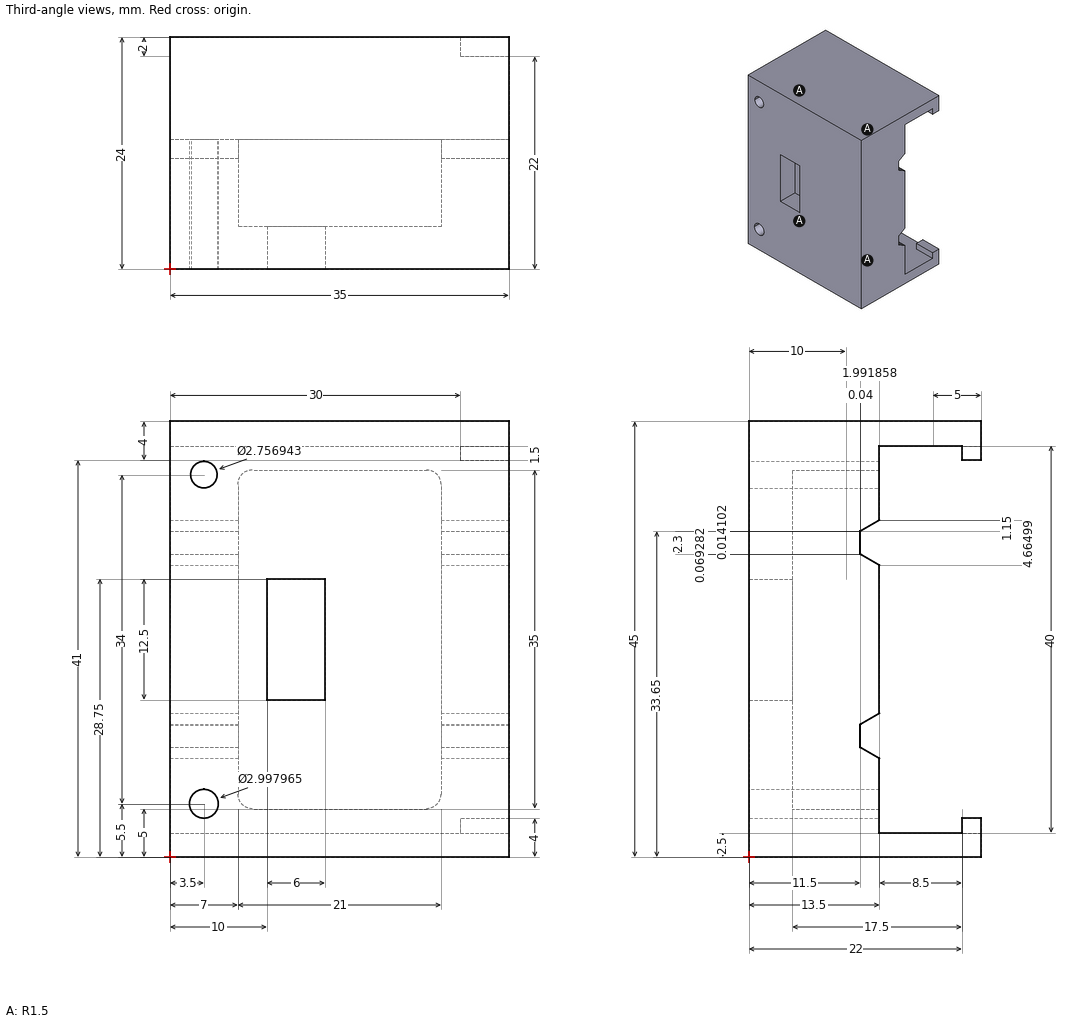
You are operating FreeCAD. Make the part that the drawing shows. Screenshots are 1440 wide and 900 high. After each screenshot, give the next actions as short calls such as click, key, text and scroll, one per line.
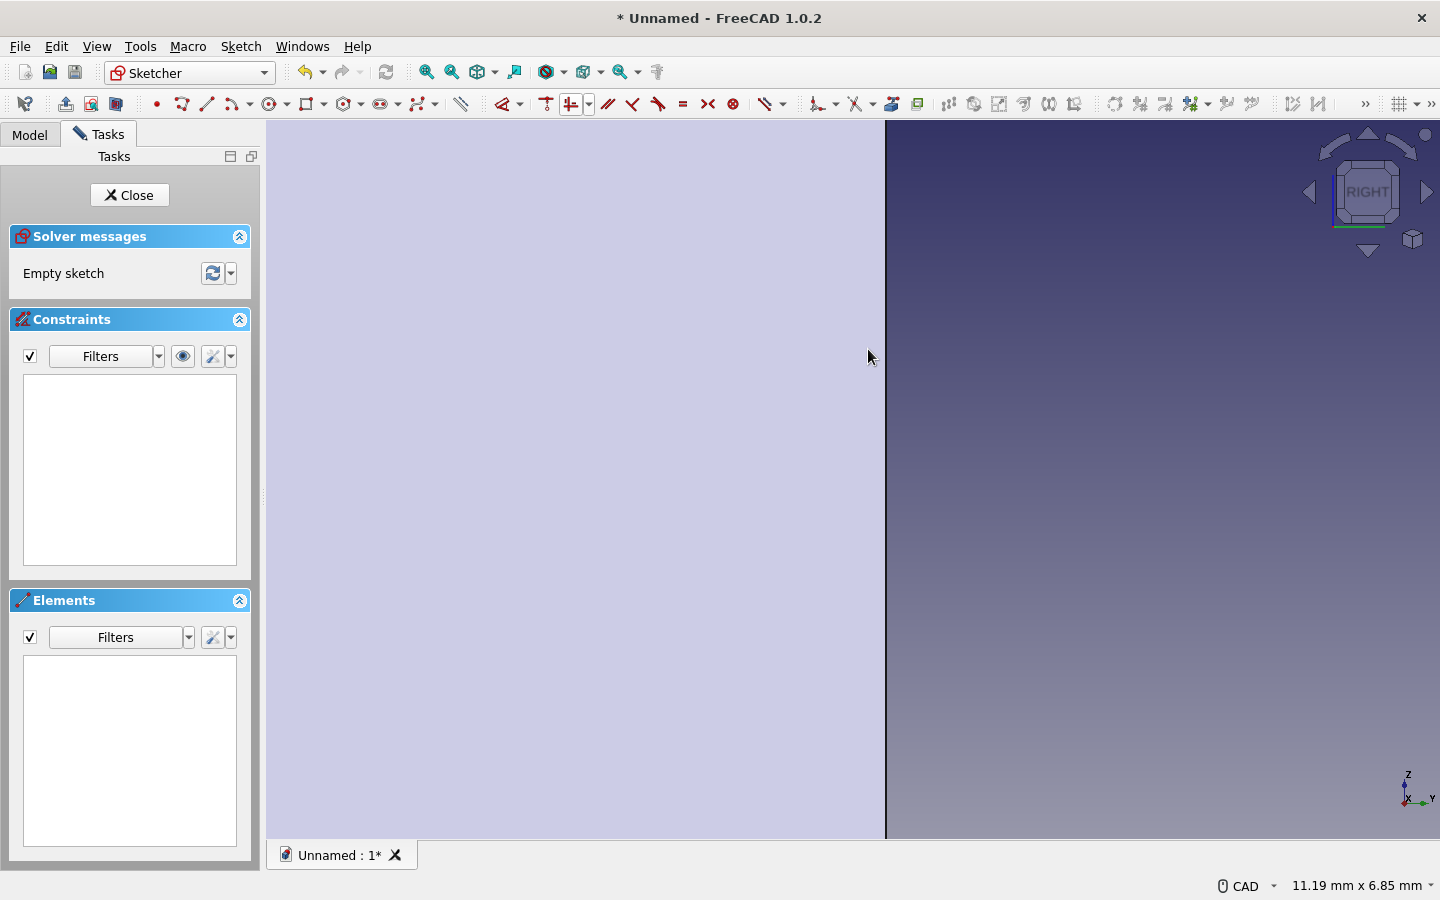
key(g)
key(m)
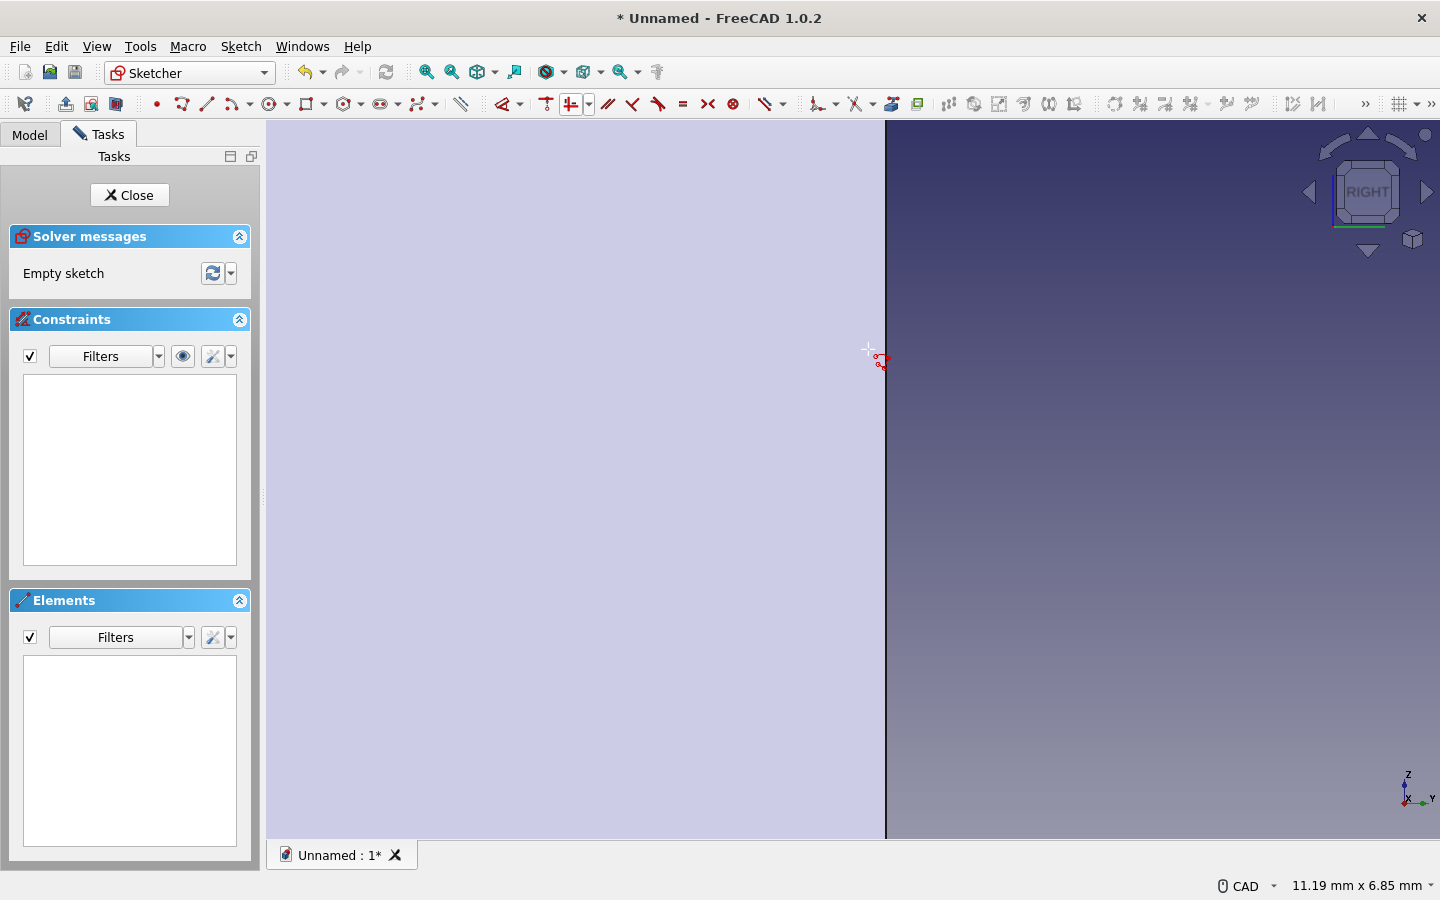
click(886, 722)
click(886, 232)
click(677, 353)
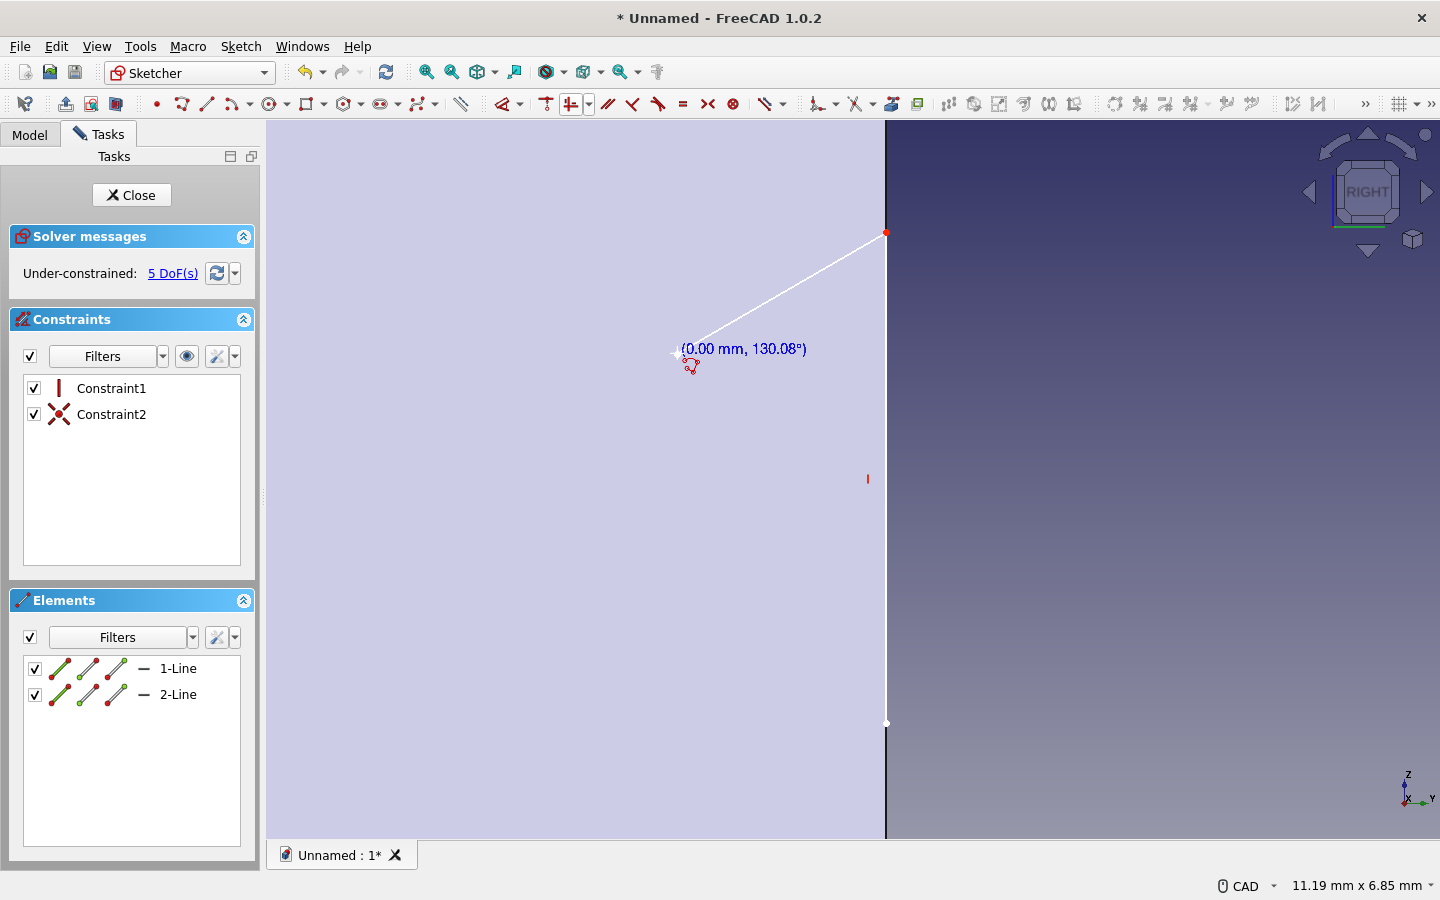
scroll(676, 354, up, 12)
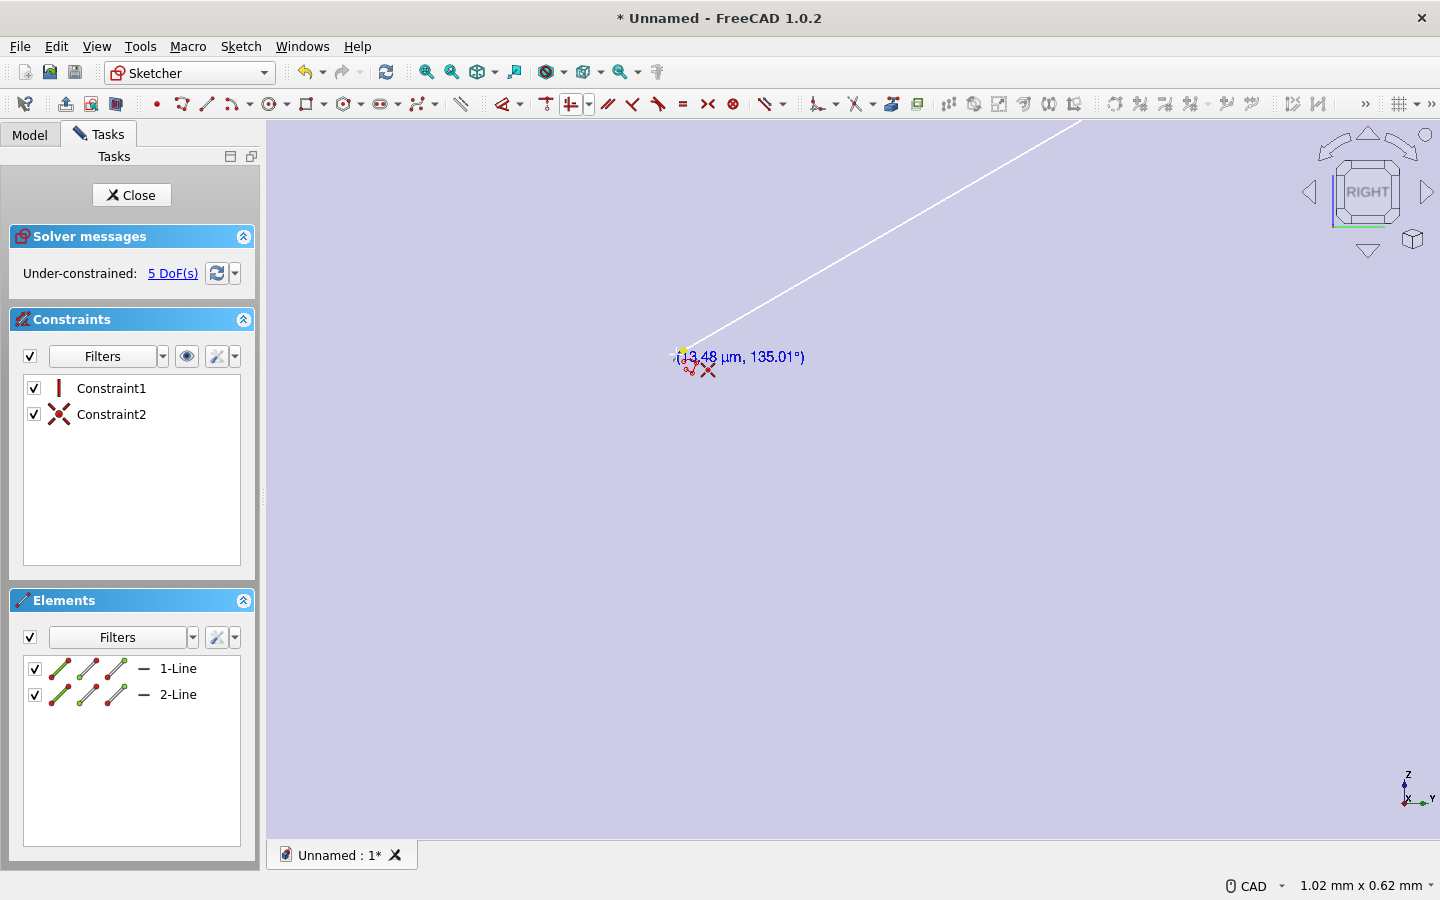
click(673, 356)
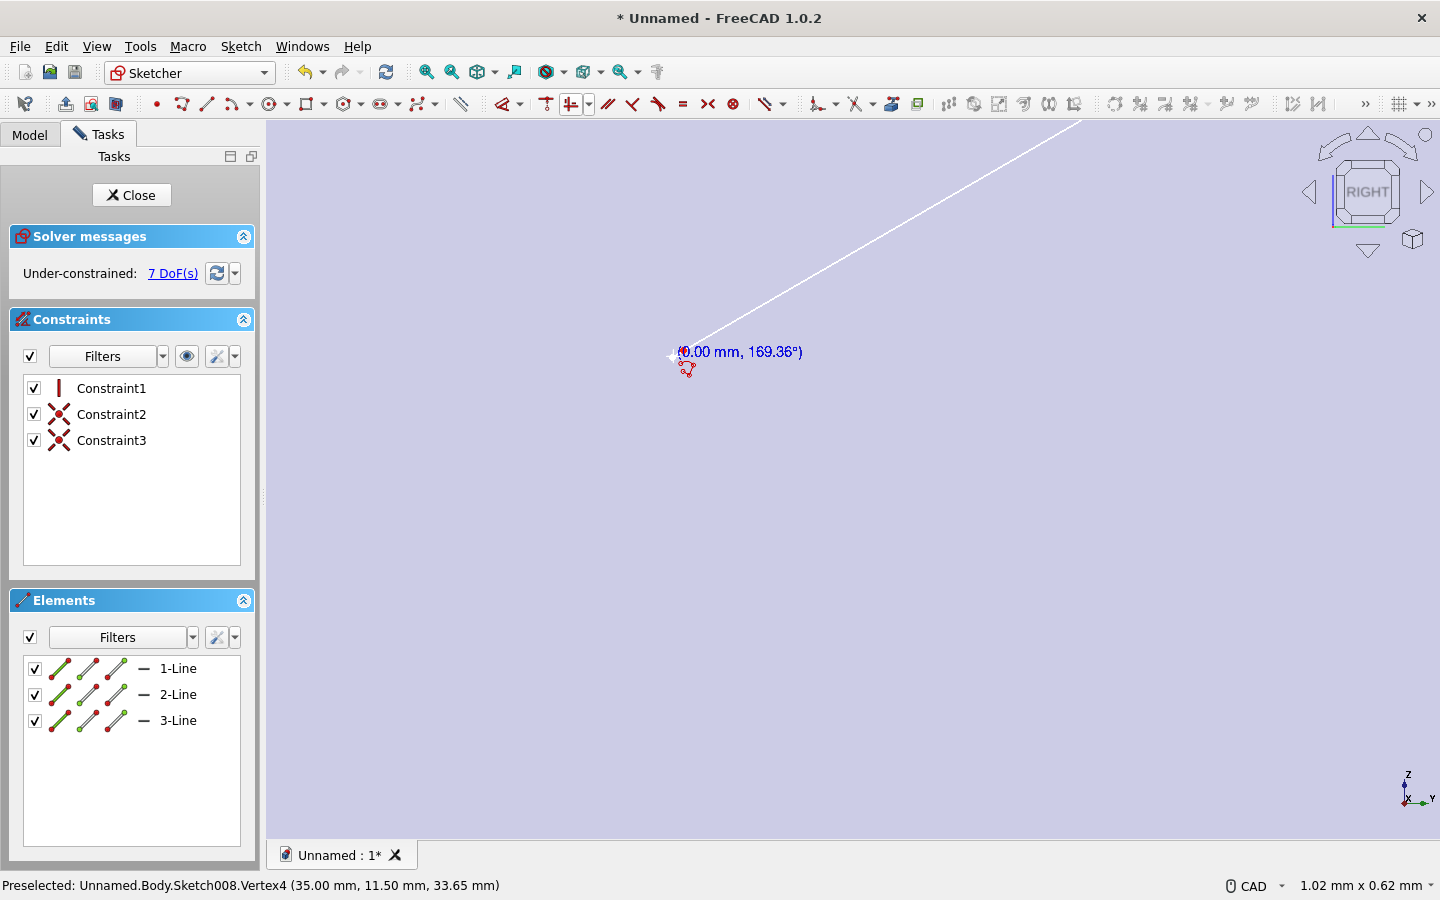
scroll(680, 357, down, 12)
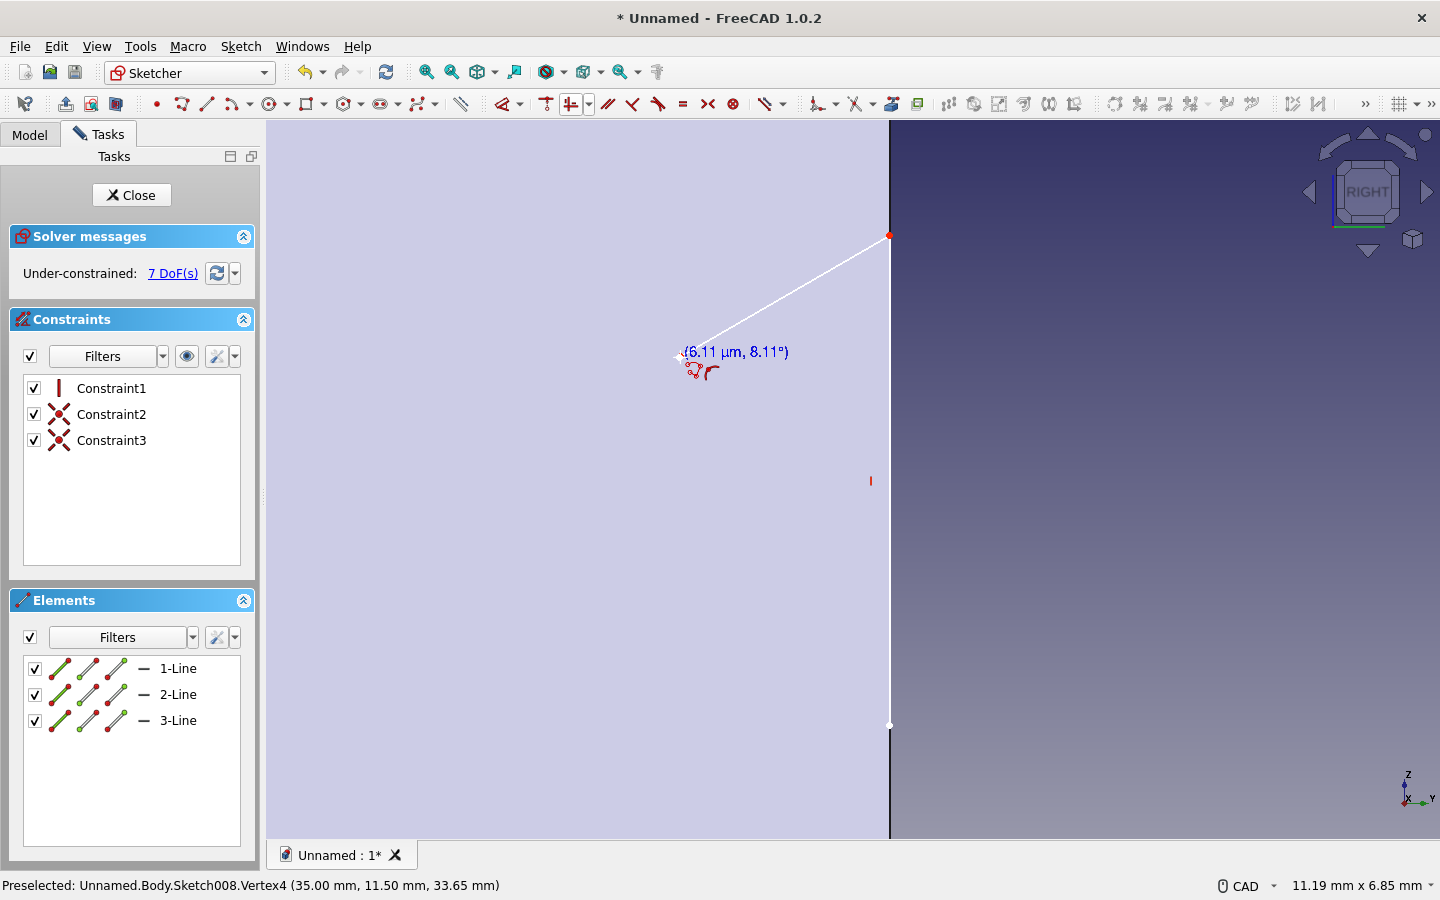
click(680, 599)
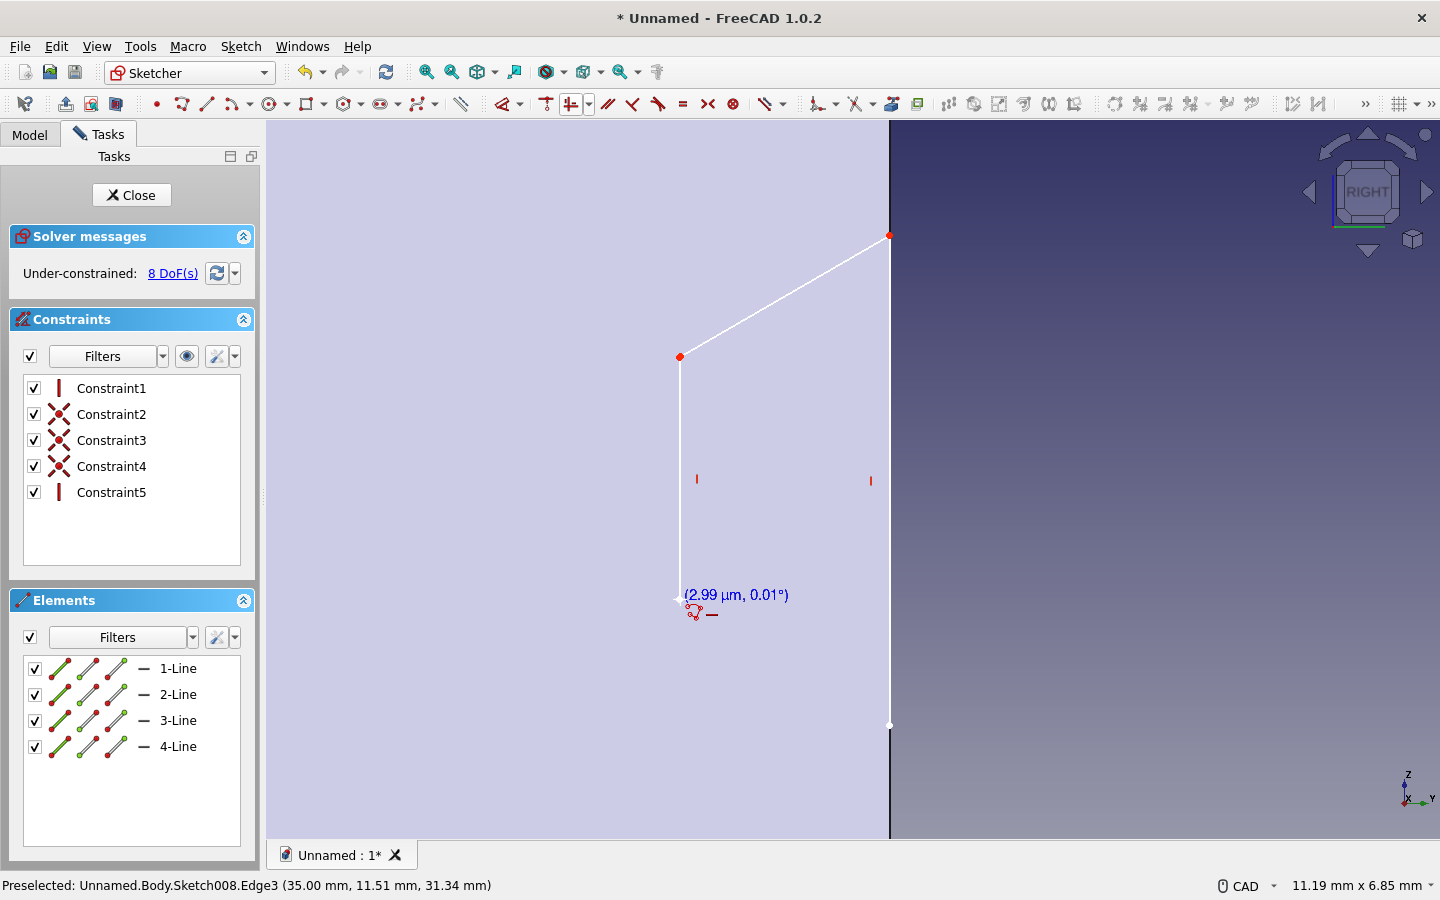
scroll(684, 606, up, 4)